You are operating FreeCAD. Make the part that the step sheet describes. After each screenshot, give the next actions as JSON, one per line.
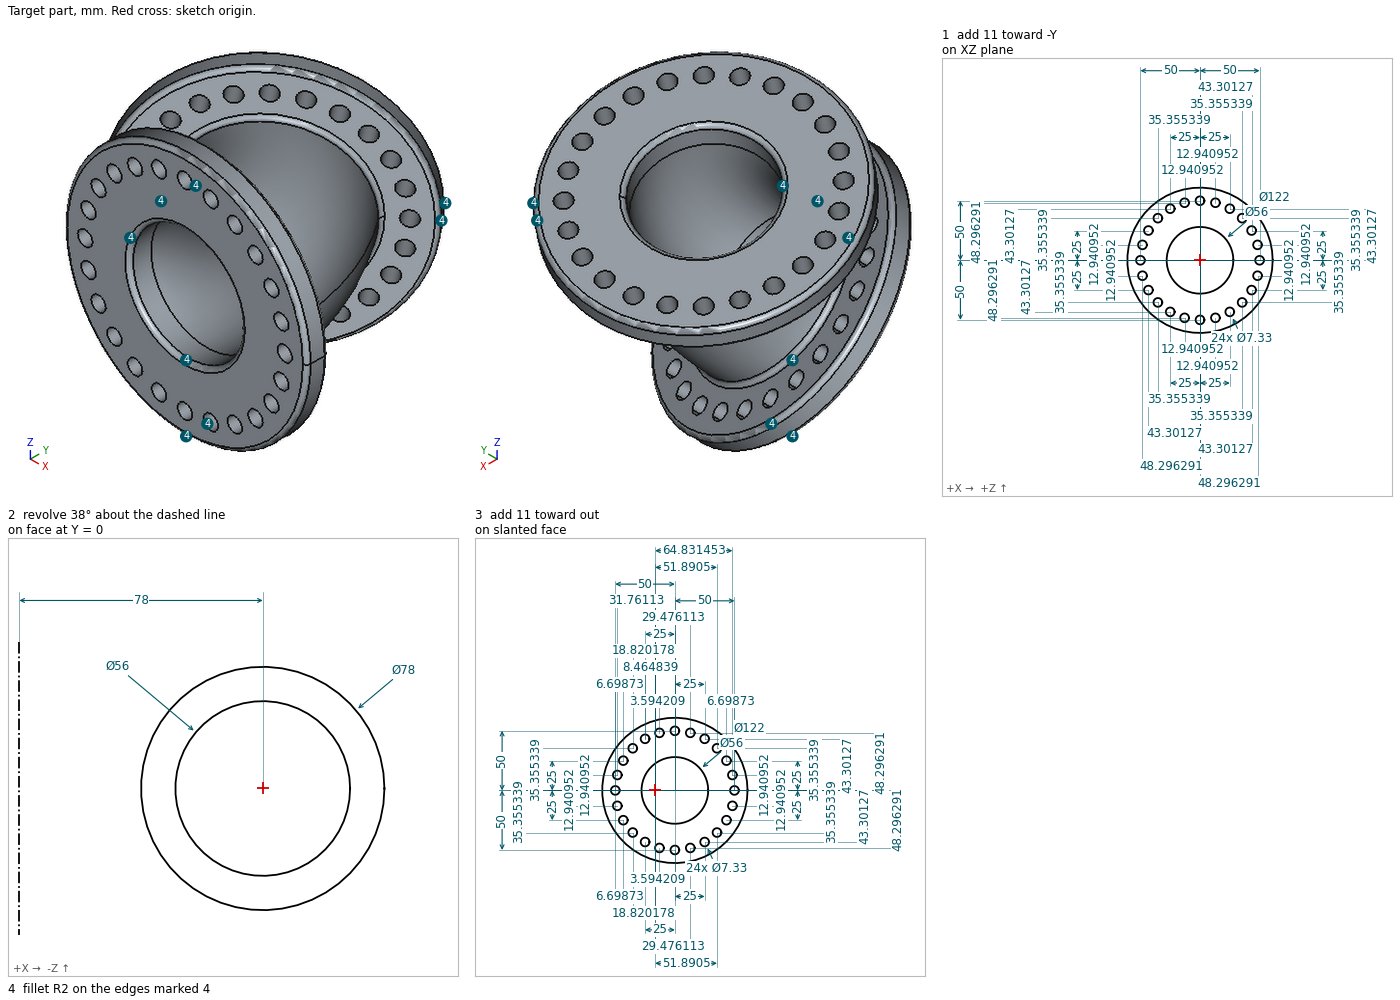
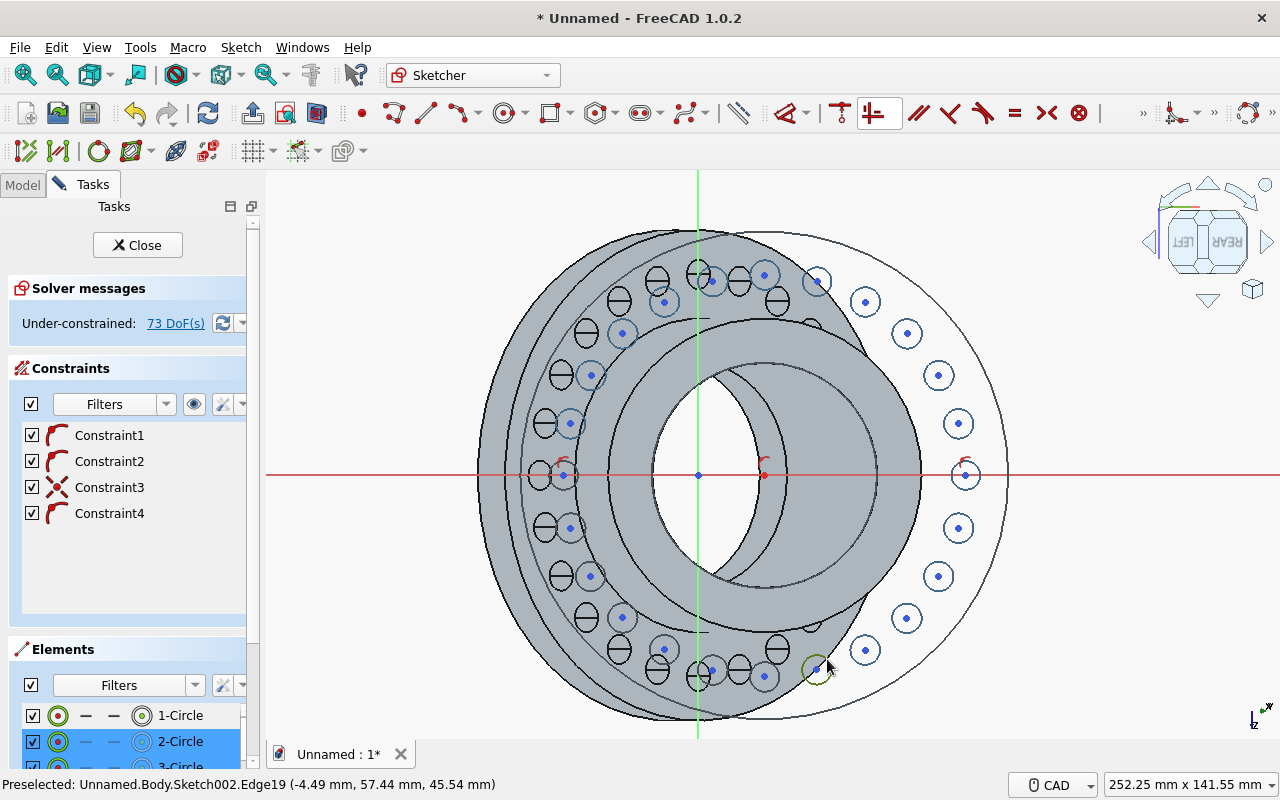
{"action": "left_click", "coordinate": [775, 667]}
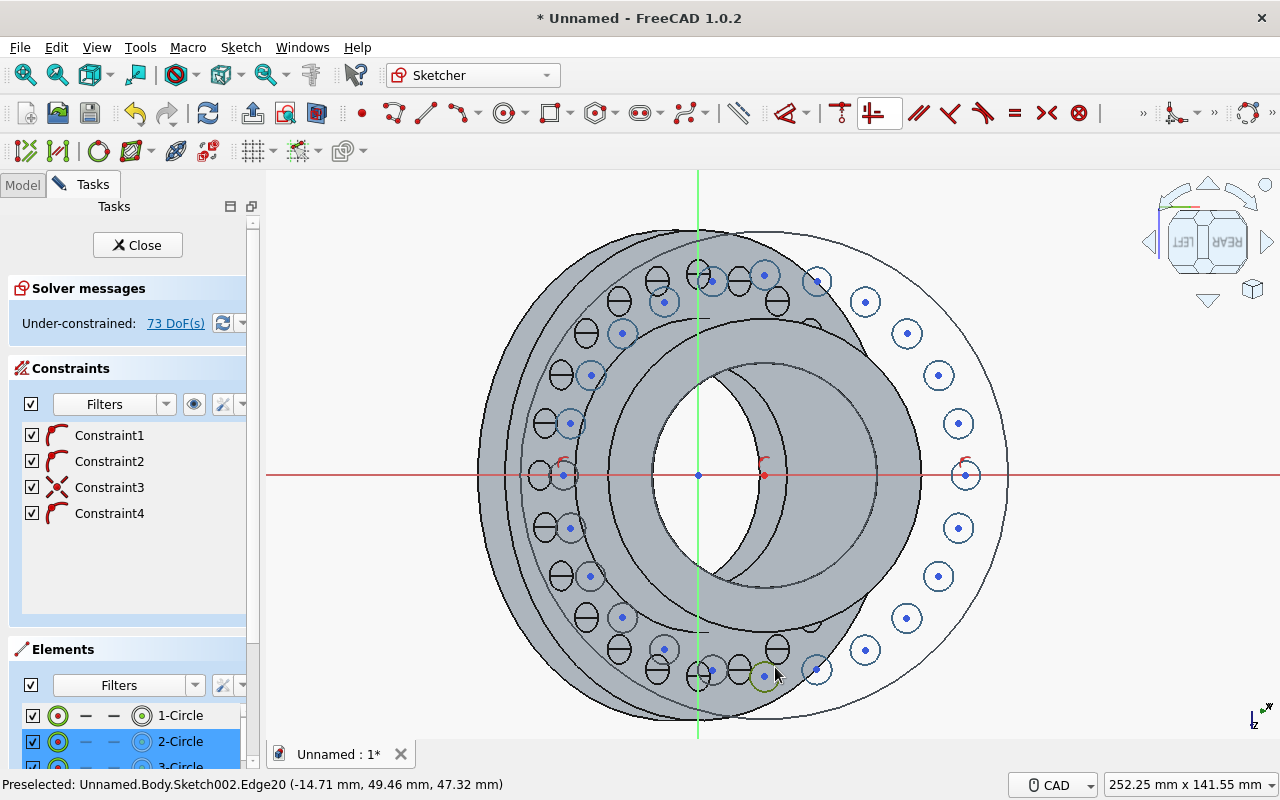
{"action": "scroll", "coordinate": [574, 465], "scroll_direction": "up", "scroll_amount": 2}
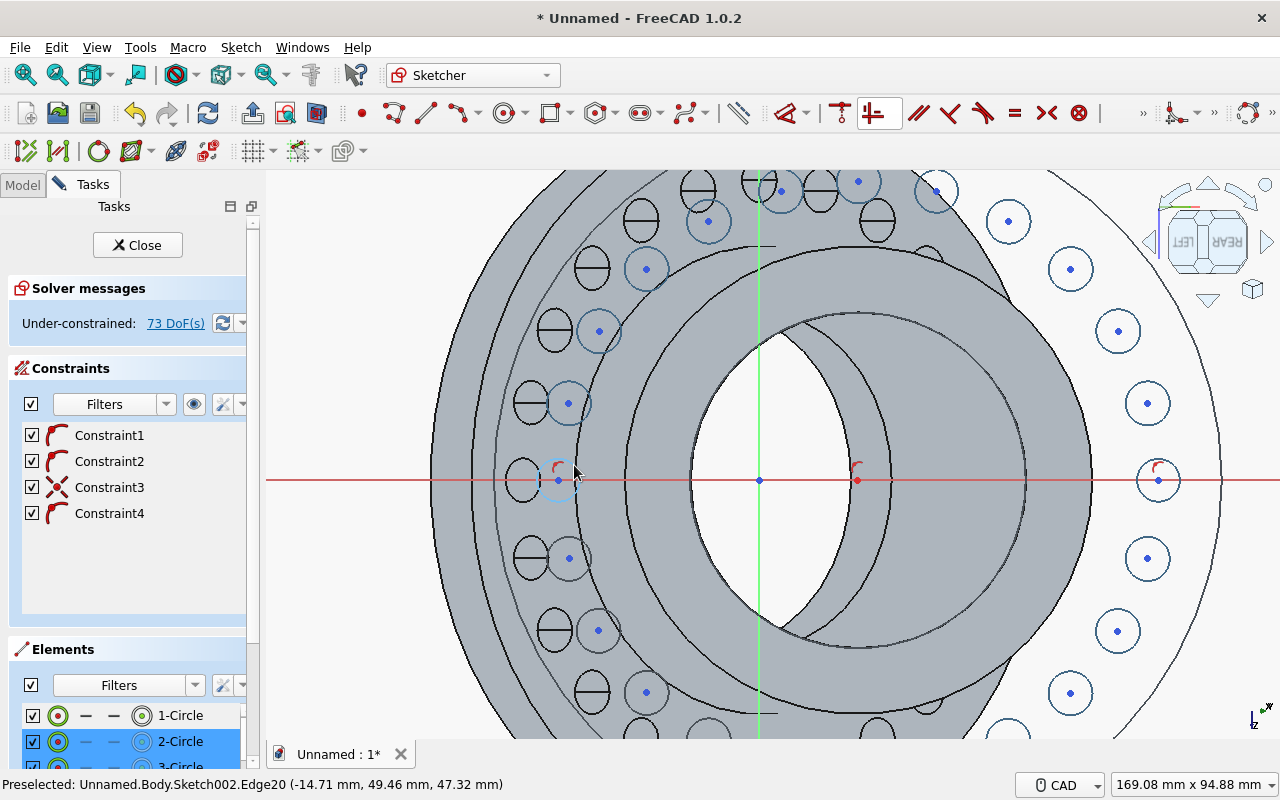
{"action": "left_click", "coordinate": [574, 465]}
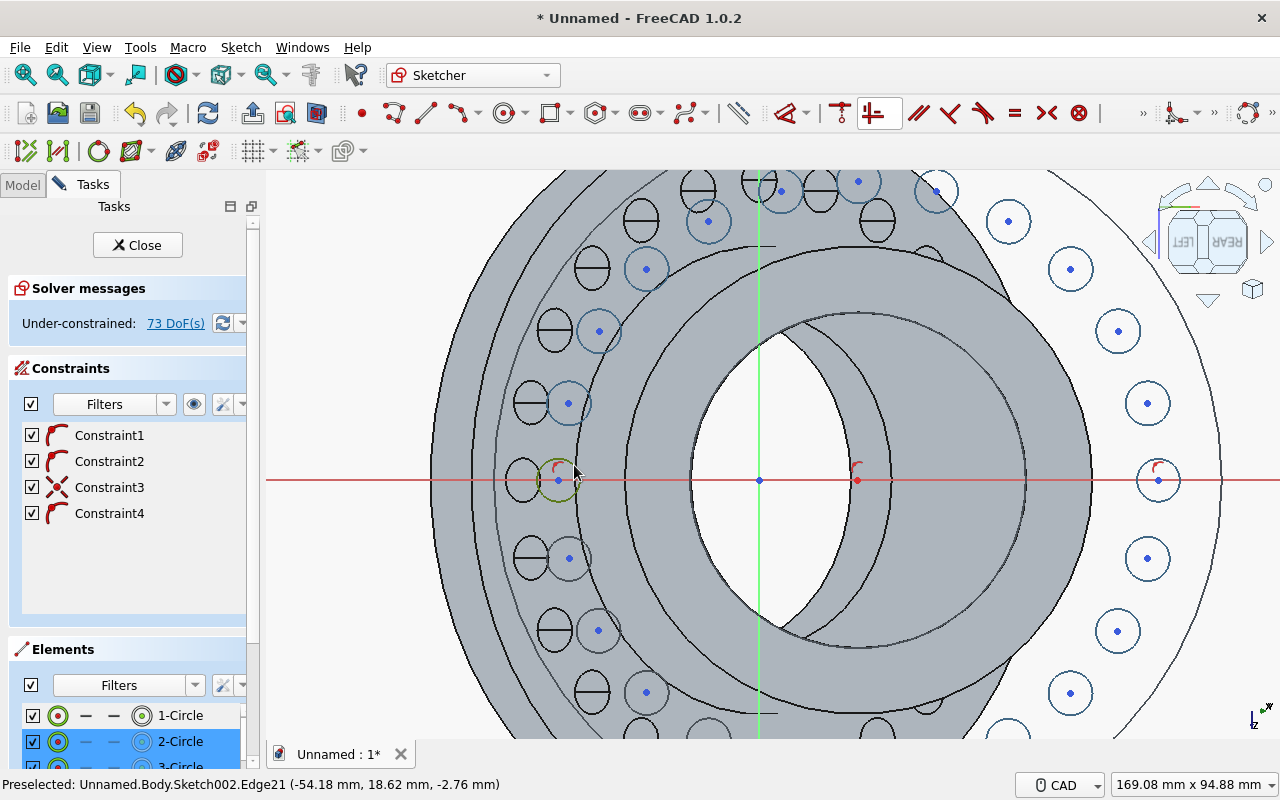
{"action": "left_click", "coordinate": [585, 543]}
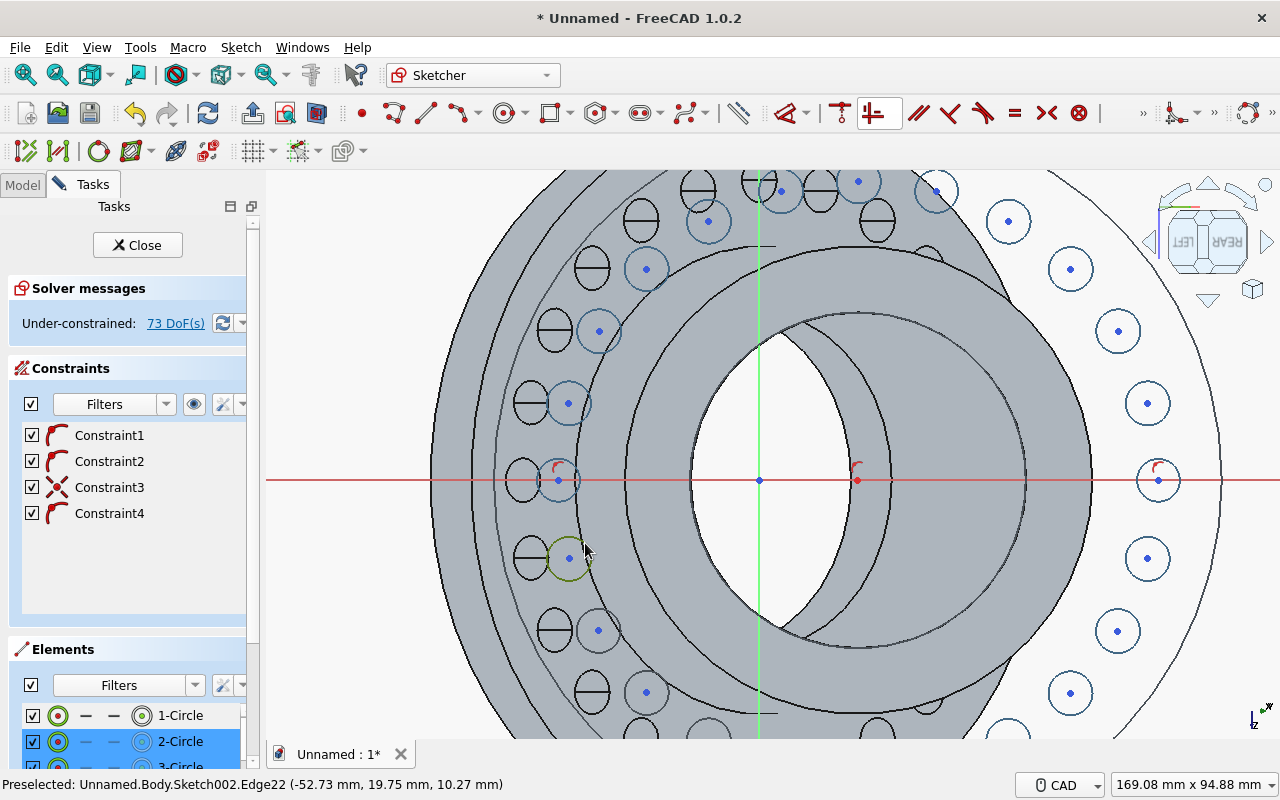
{"action": "left_click", "coordinate": [614, 615]}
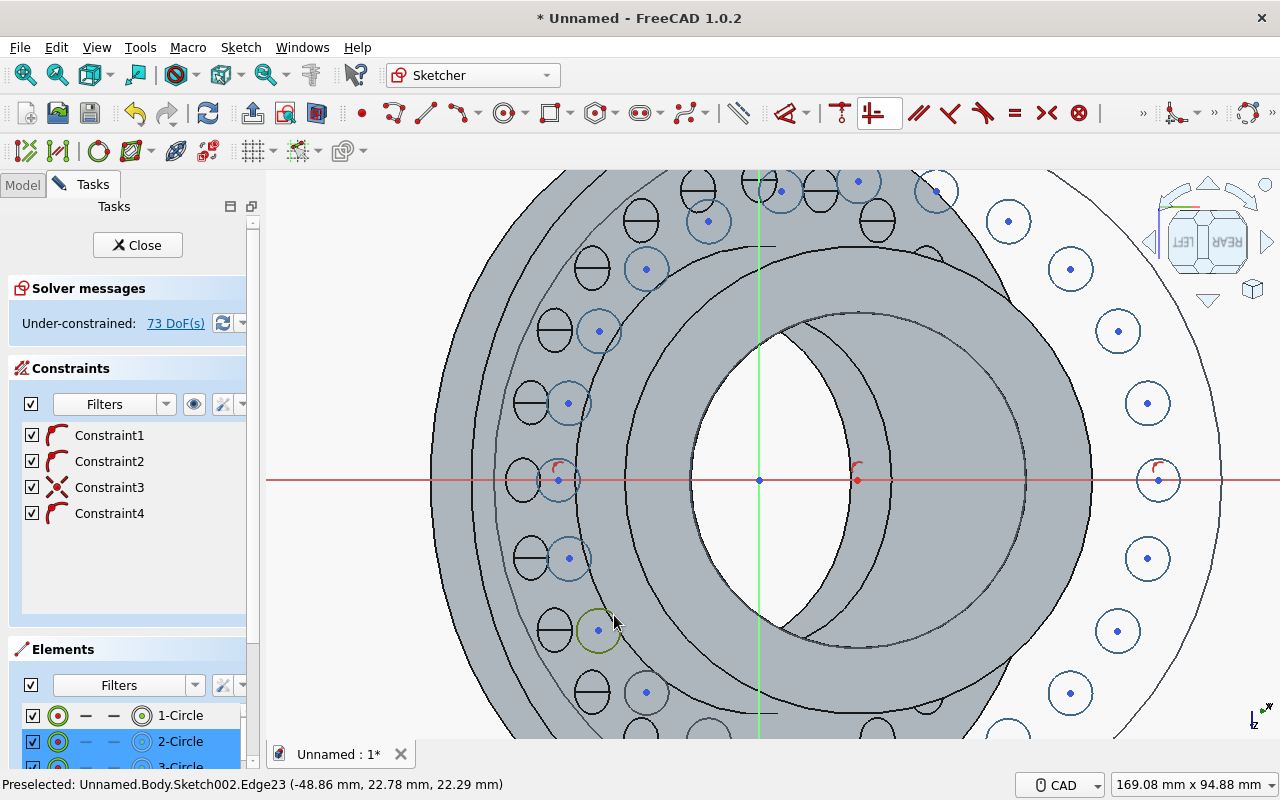
{"action": "scroll", "coordinate": [579, 433], "scroll_direction": "down", "scroll_amount": 4}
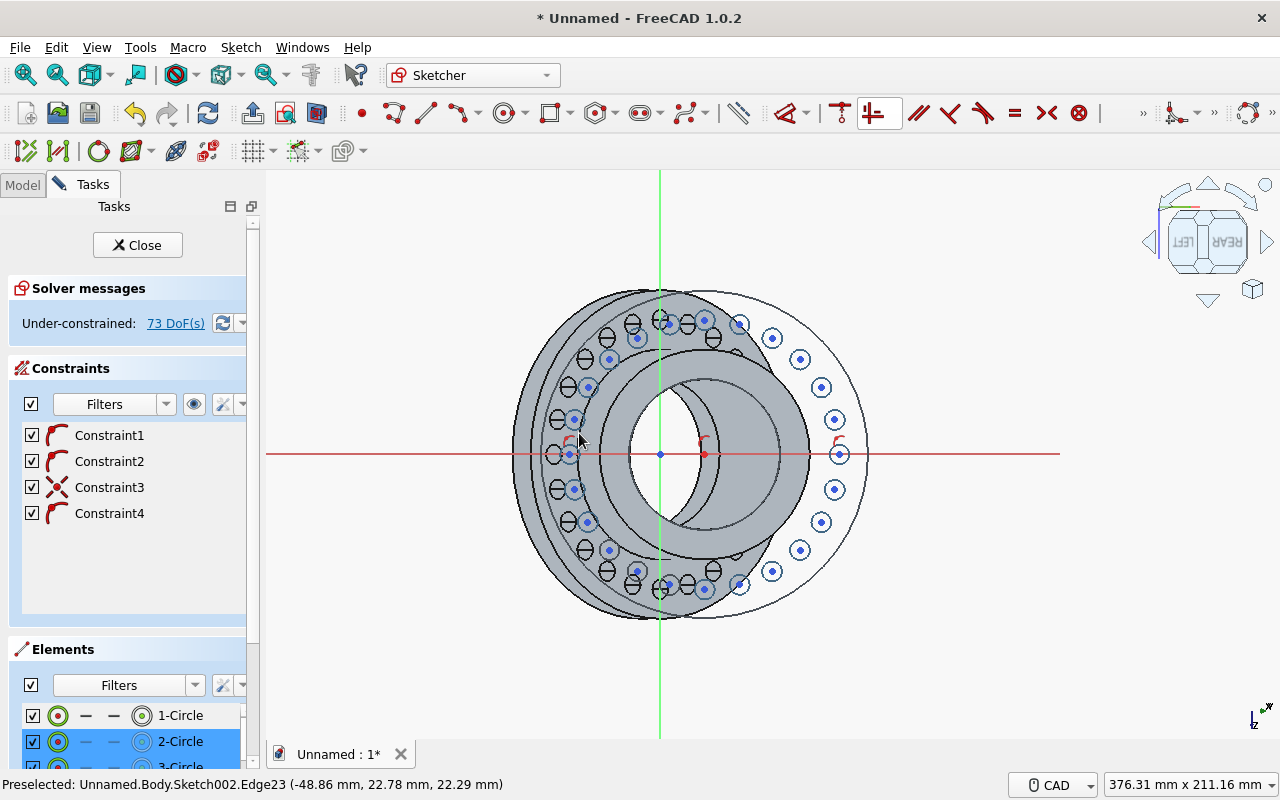
{"action": "scroll", "coordinate": [677, 578], "scroll_direction": "up", "scroll_amount": 2}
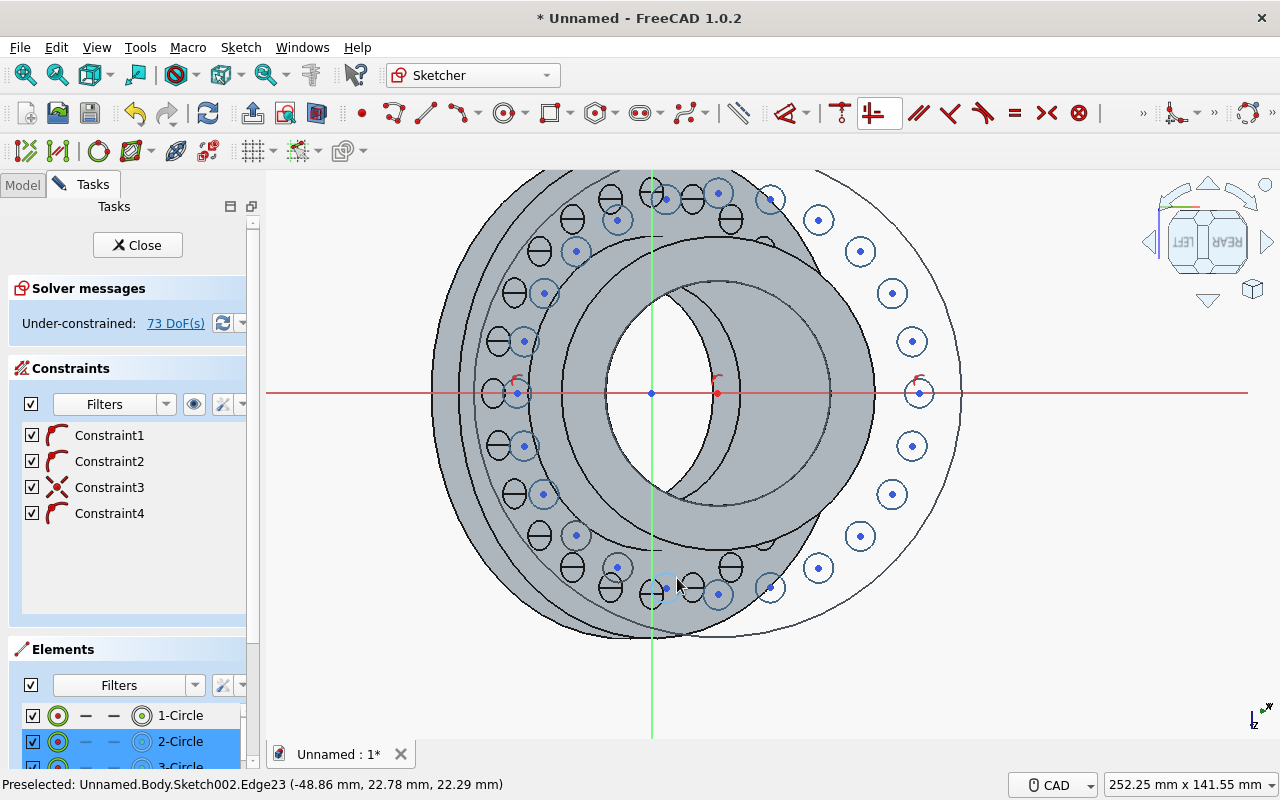
{"action": "left_click", "coordinate": [677, 578]}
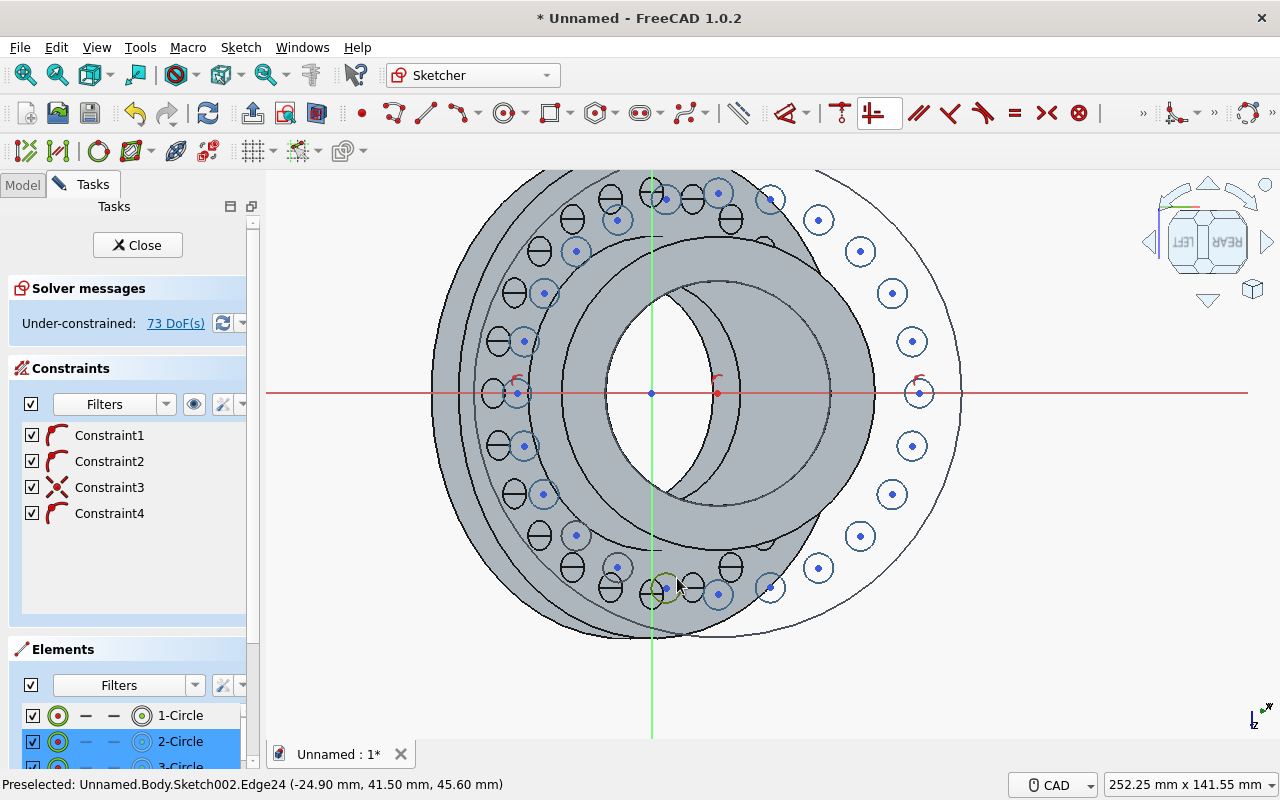
{"action": "left_click", "coordinate": [628, 557]}